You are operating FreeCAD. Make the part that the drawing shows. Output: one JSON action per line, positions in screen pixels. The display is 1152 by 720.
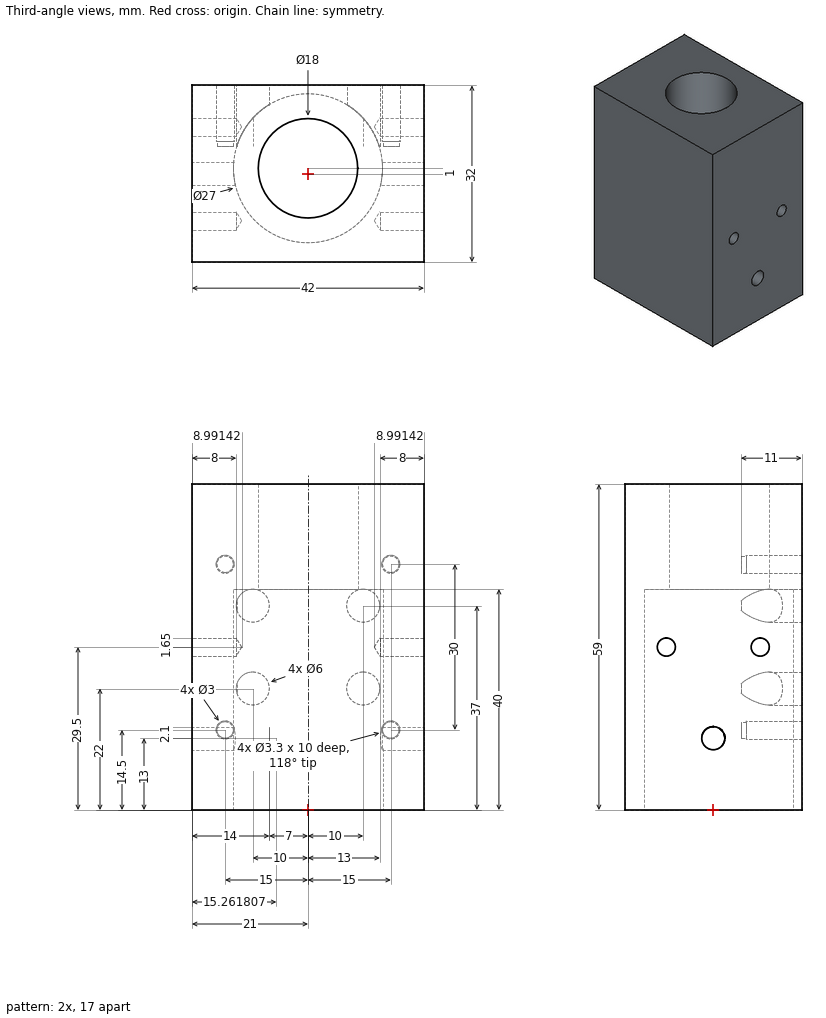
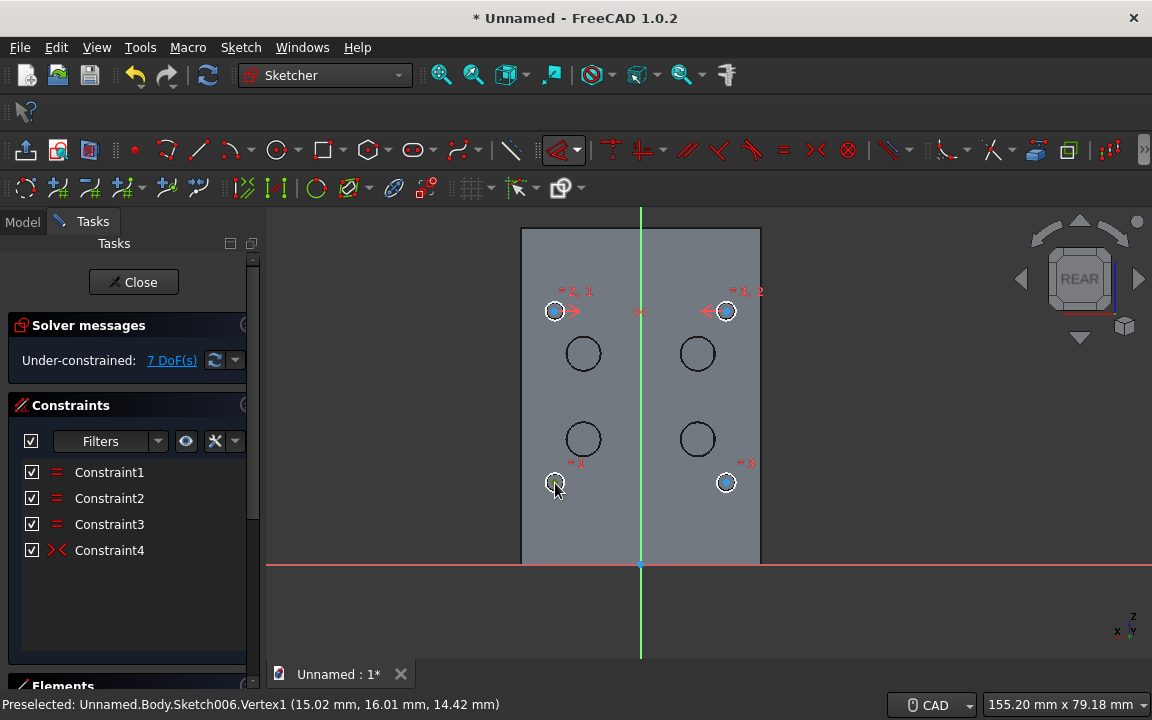
{"action": "left_click", "coordinate": [726, 483]}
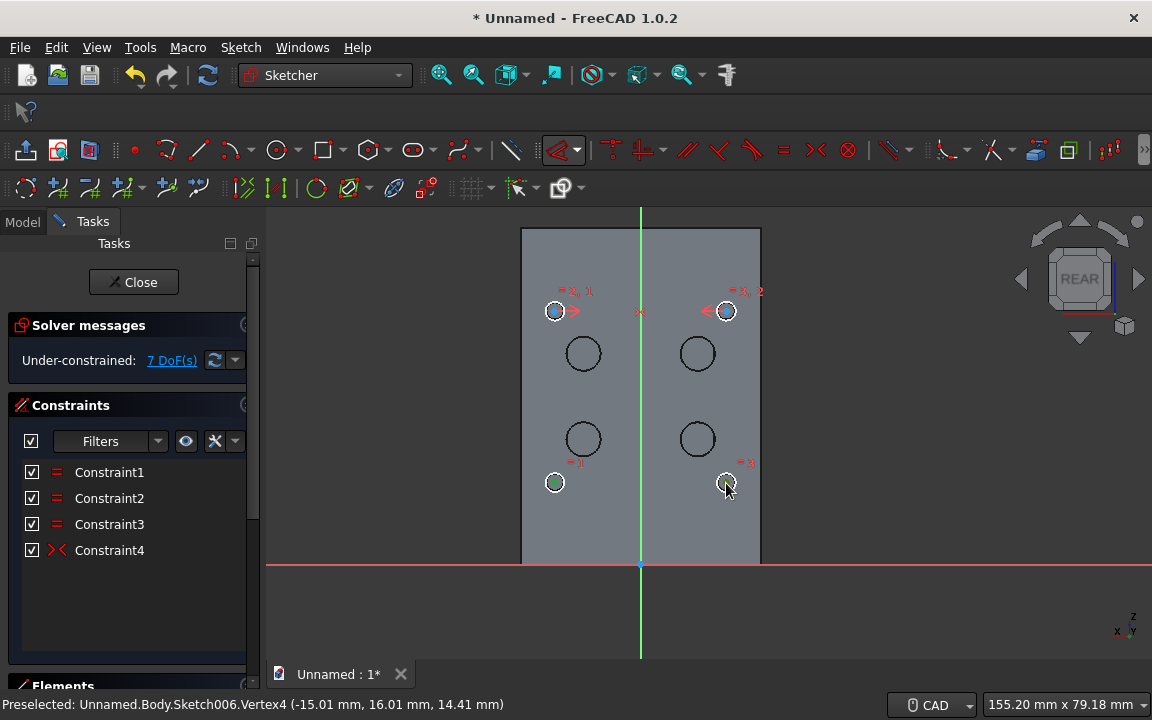
{"action": "left_click", "coordinate": [641, 603]}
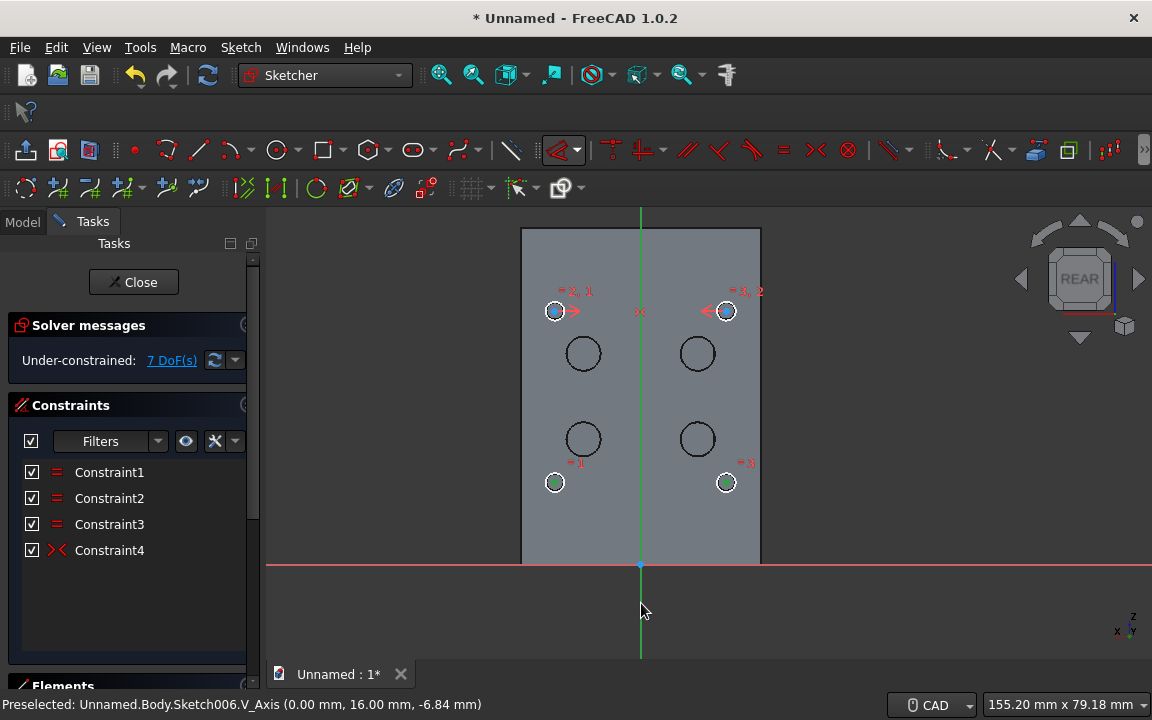
{"action": "key", "text": "s"}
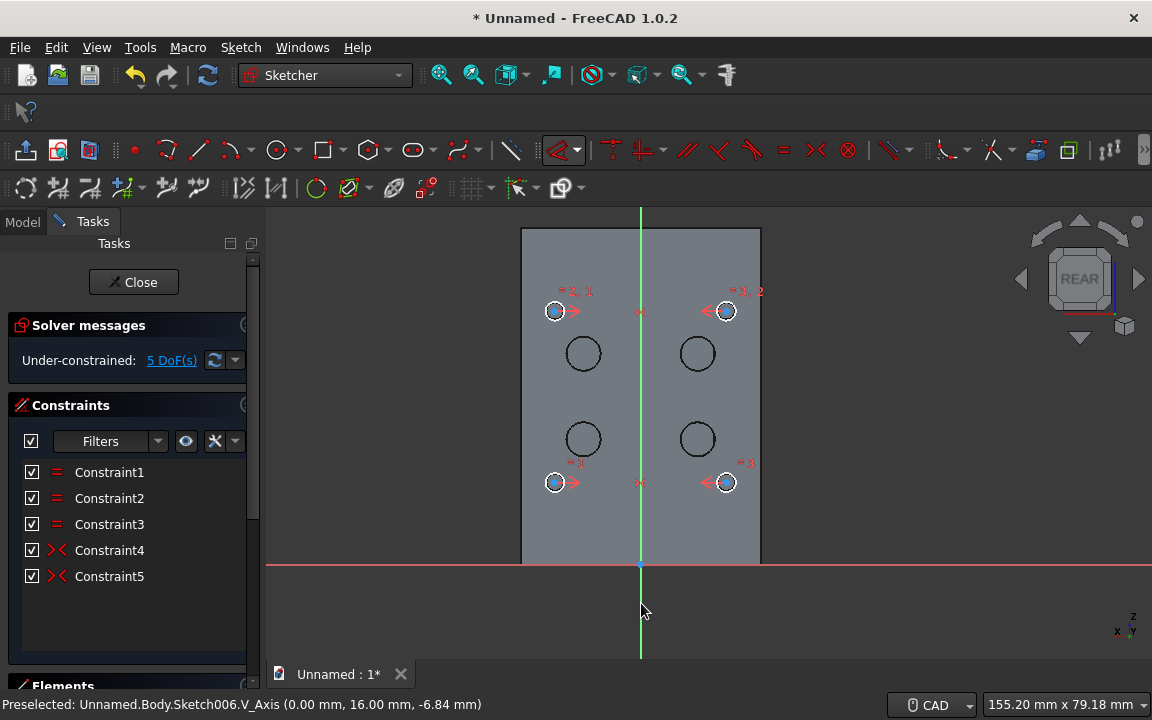
{"action": "scroll", "coordinate": [562, 476], "scroll_direction": "up", "scroll_amount": 4}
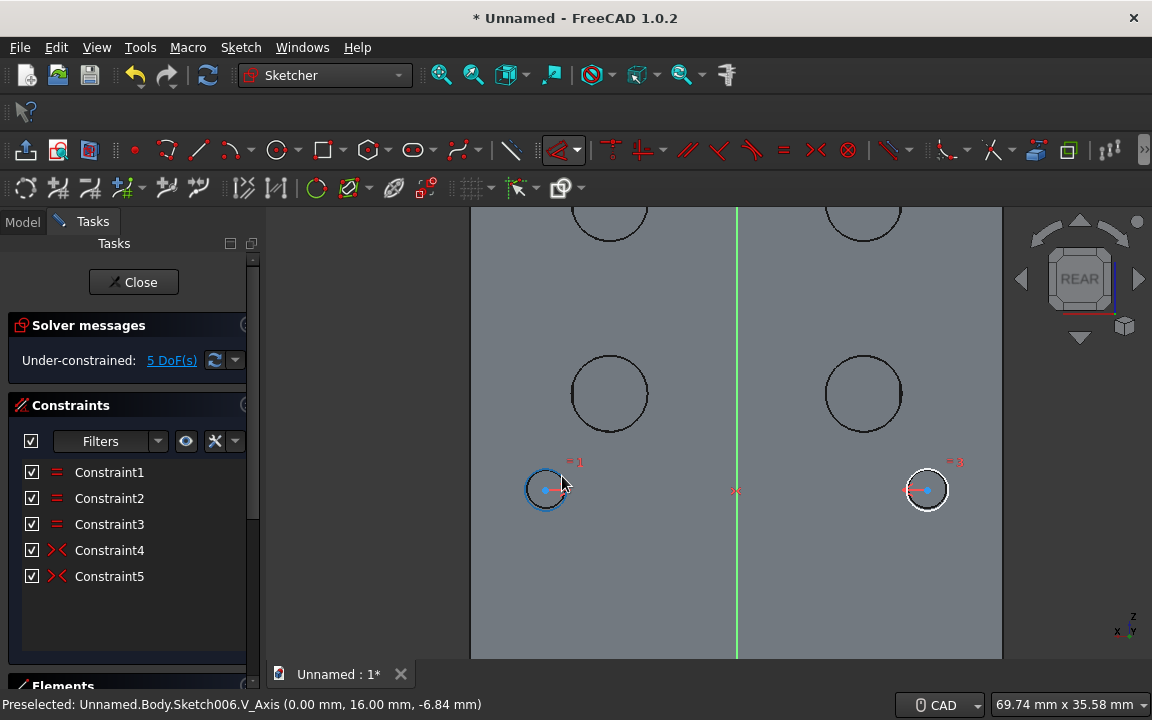
{"action": "left_click", "coordinate": [560, 475]}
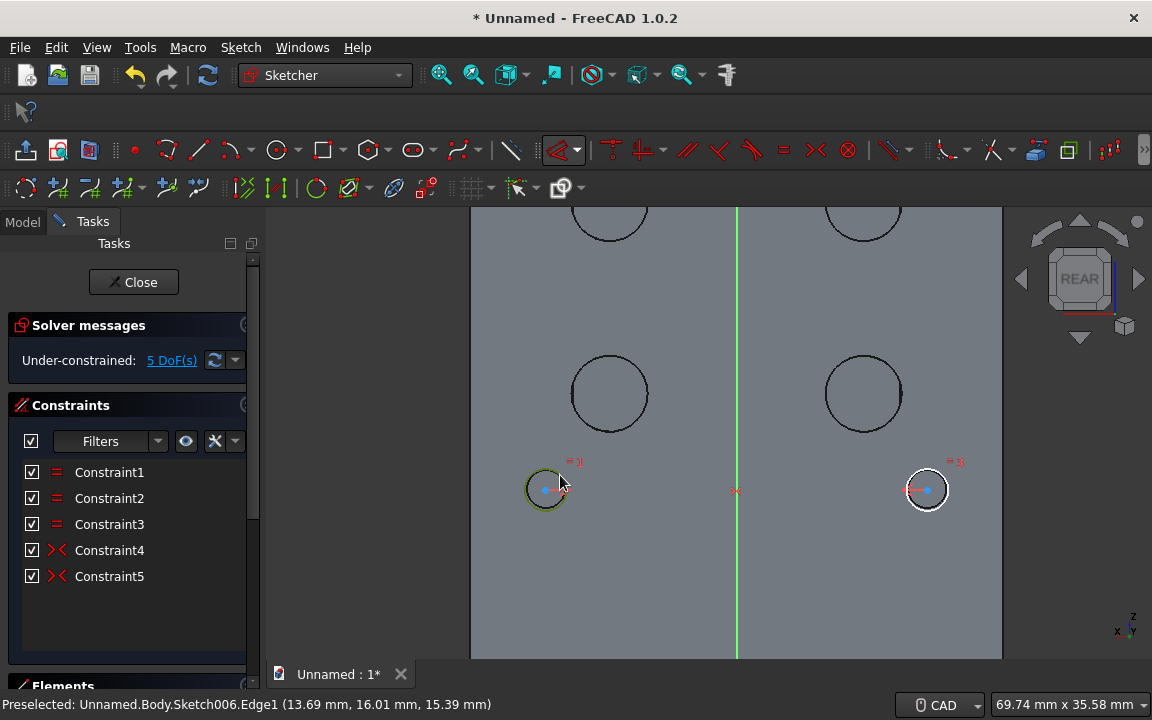
{"action": "key", "text": "k o"}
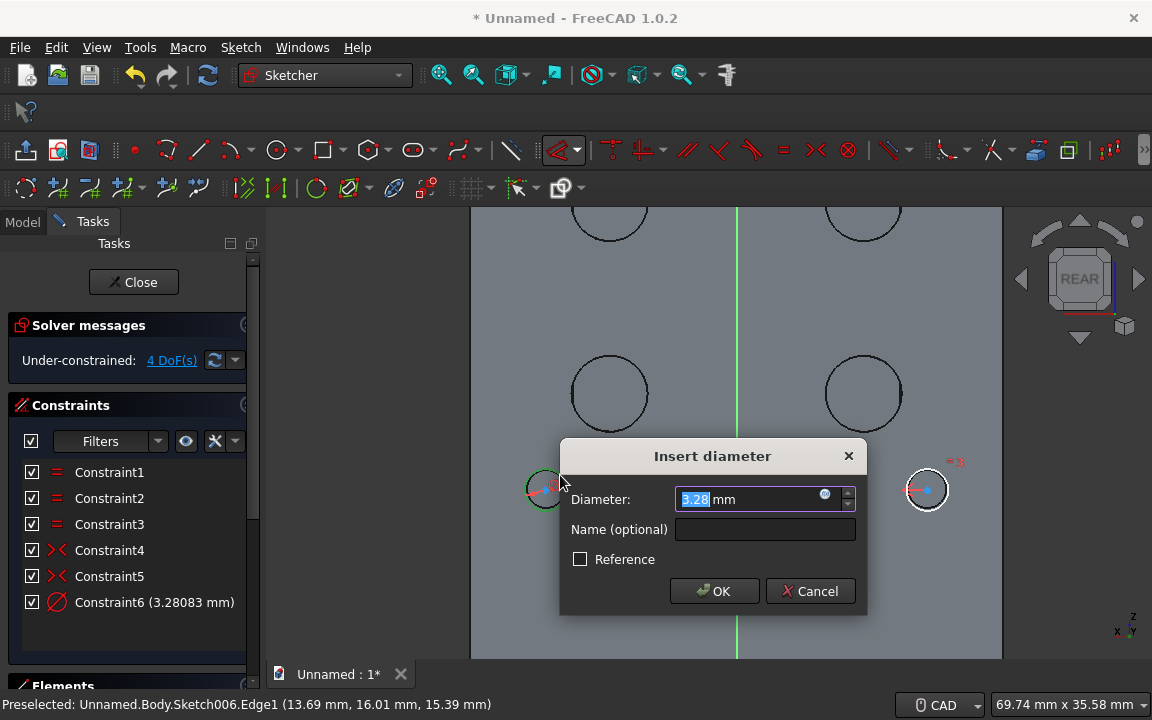
{"action": "type", "text": "3.3"}
{"action": "key", "text": "Return"}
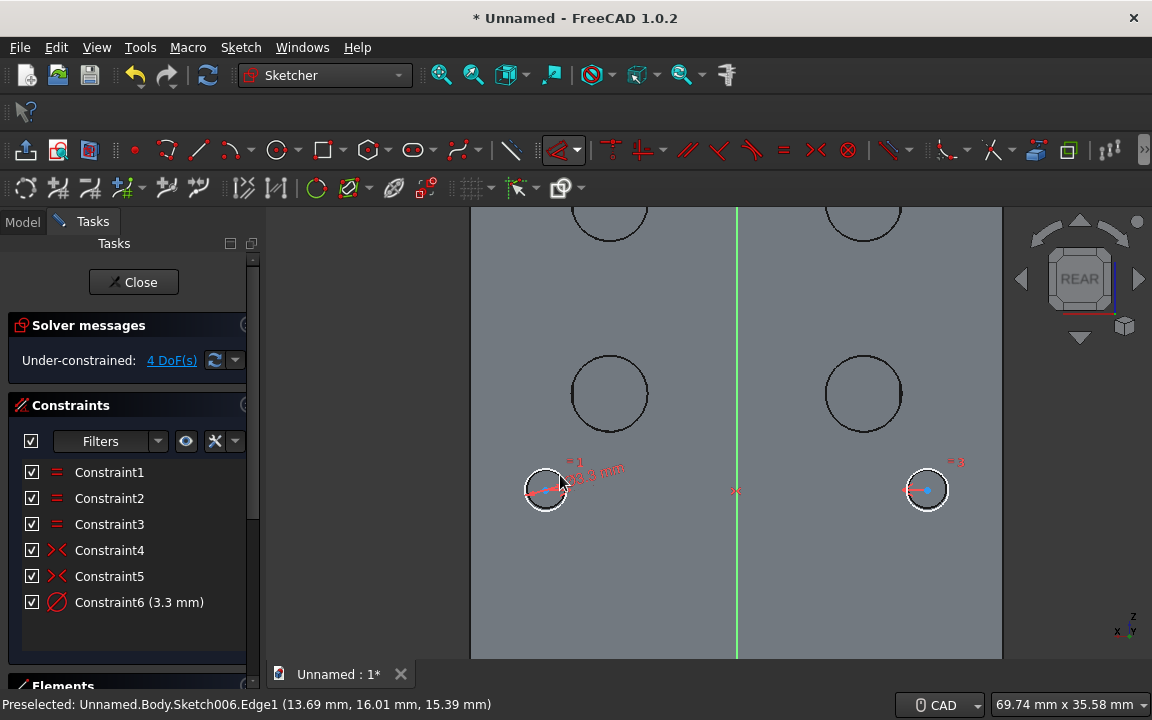
{"action": "left_click", "coordinate": [546, 490]}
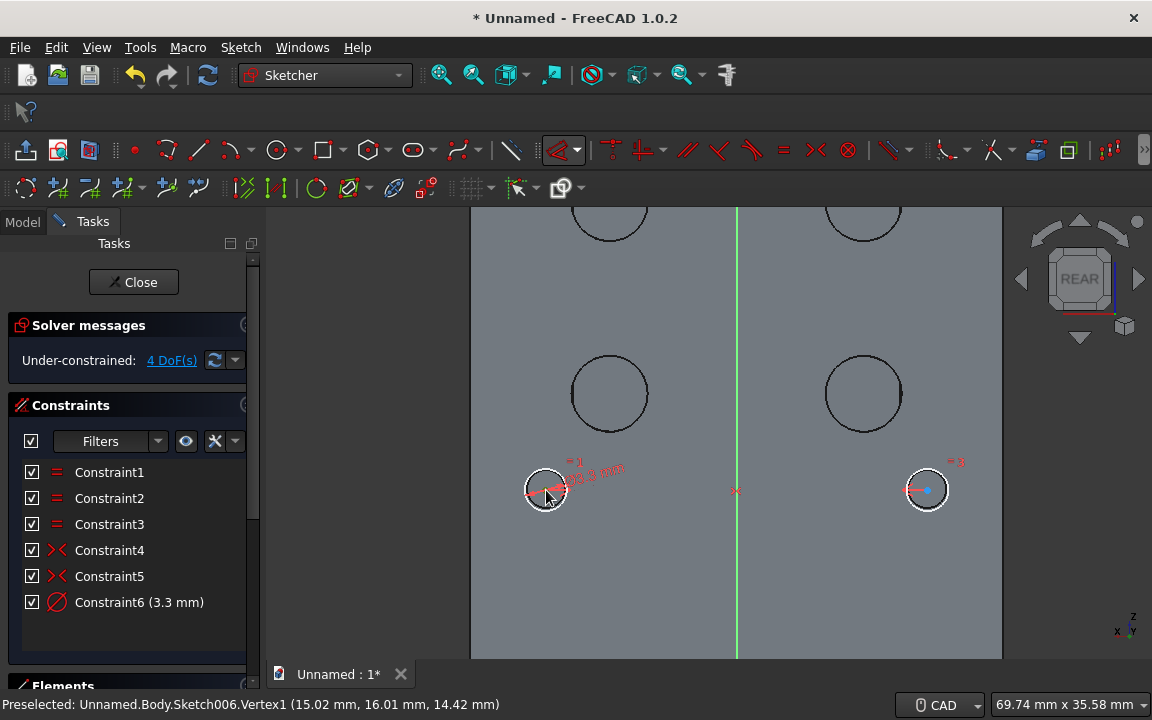
{"action": "key", "text": "l"}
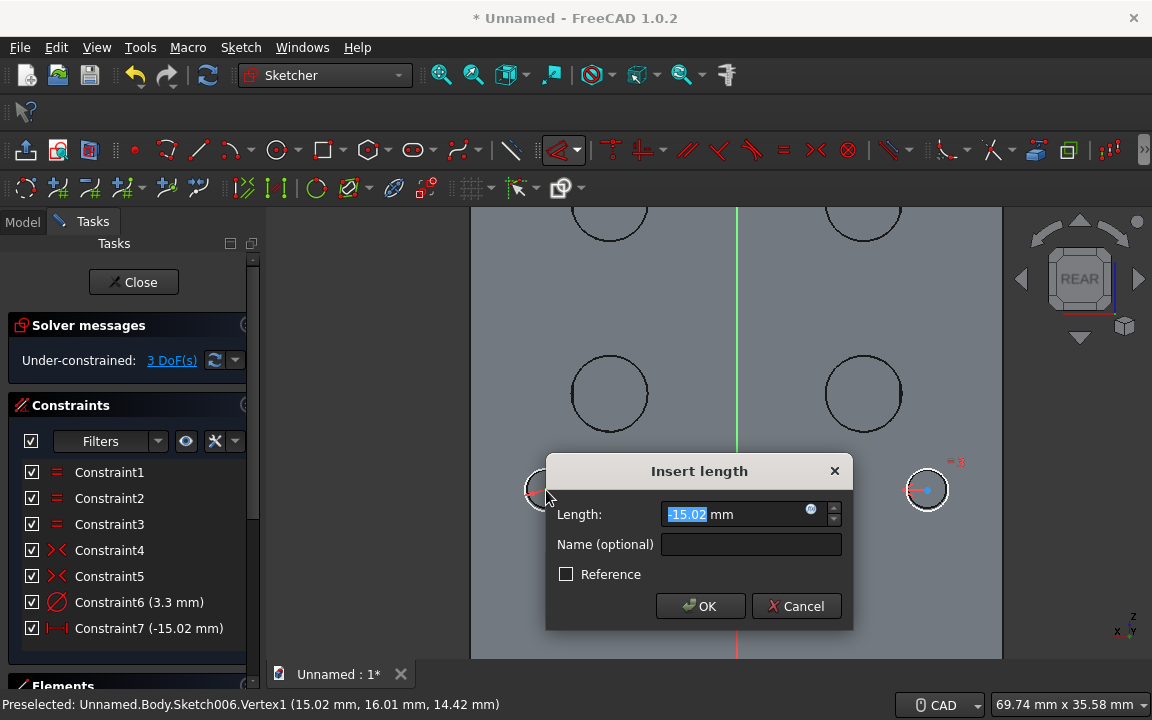
{"action": "type", "text": "-15"}
{"action": "key", "text": "Return"}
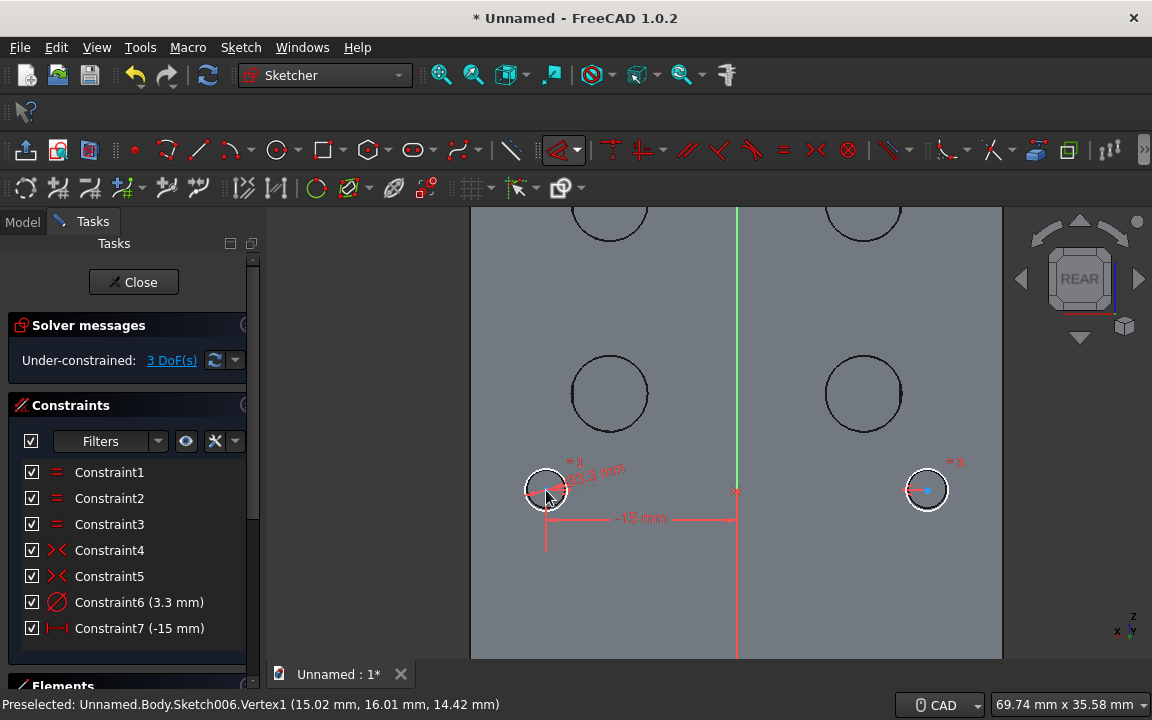
{"action": "scroll", "coordinate": [562, 476], "scroll_direction": "down", "scroll_amount": 4}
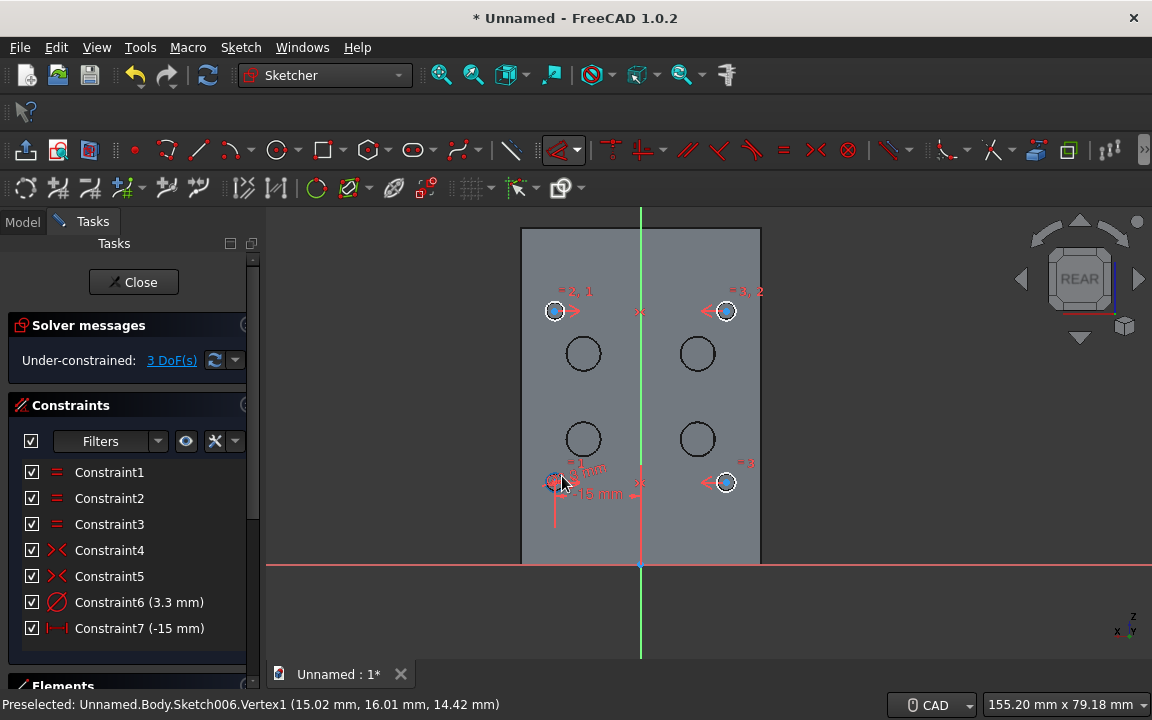
{"action": "left_click", "coordinate": [555, 311]}